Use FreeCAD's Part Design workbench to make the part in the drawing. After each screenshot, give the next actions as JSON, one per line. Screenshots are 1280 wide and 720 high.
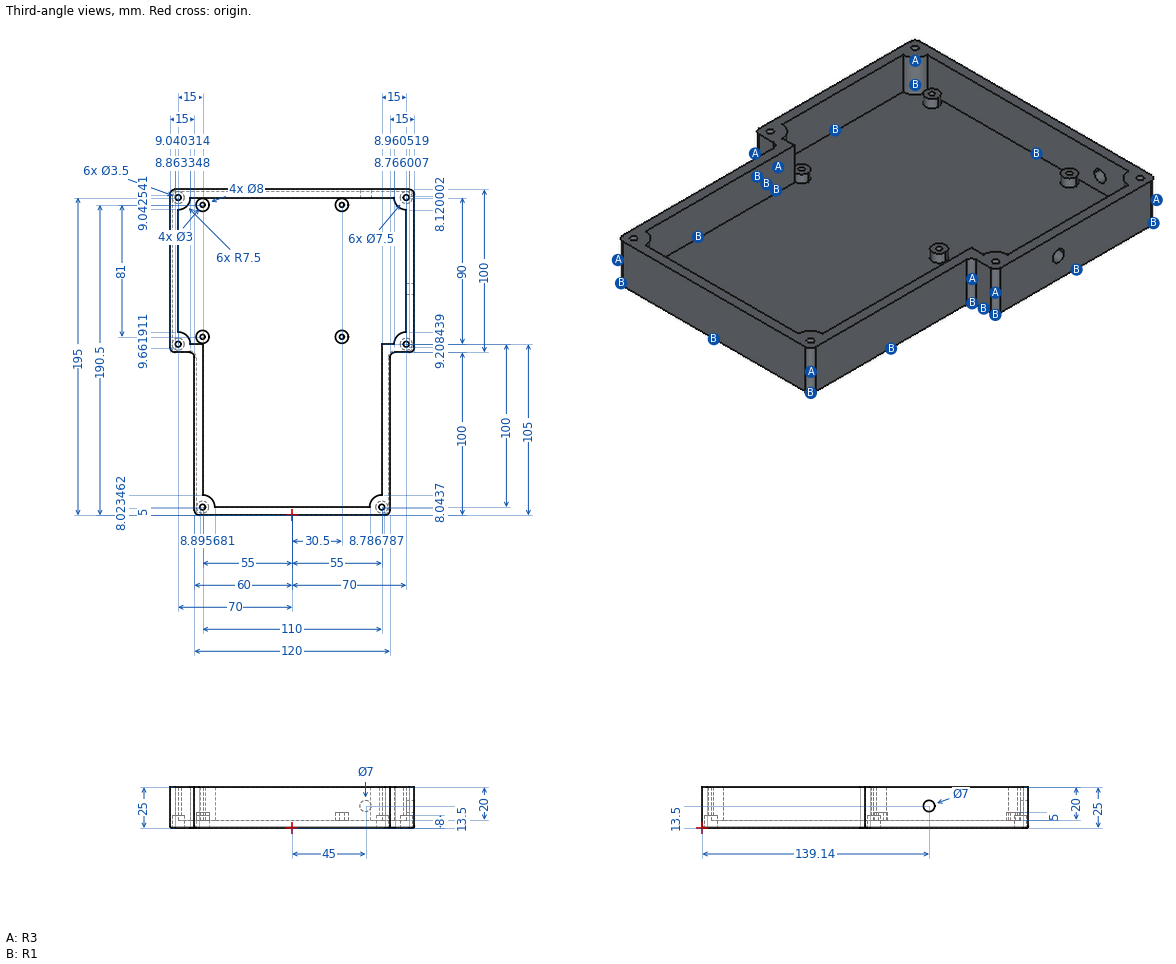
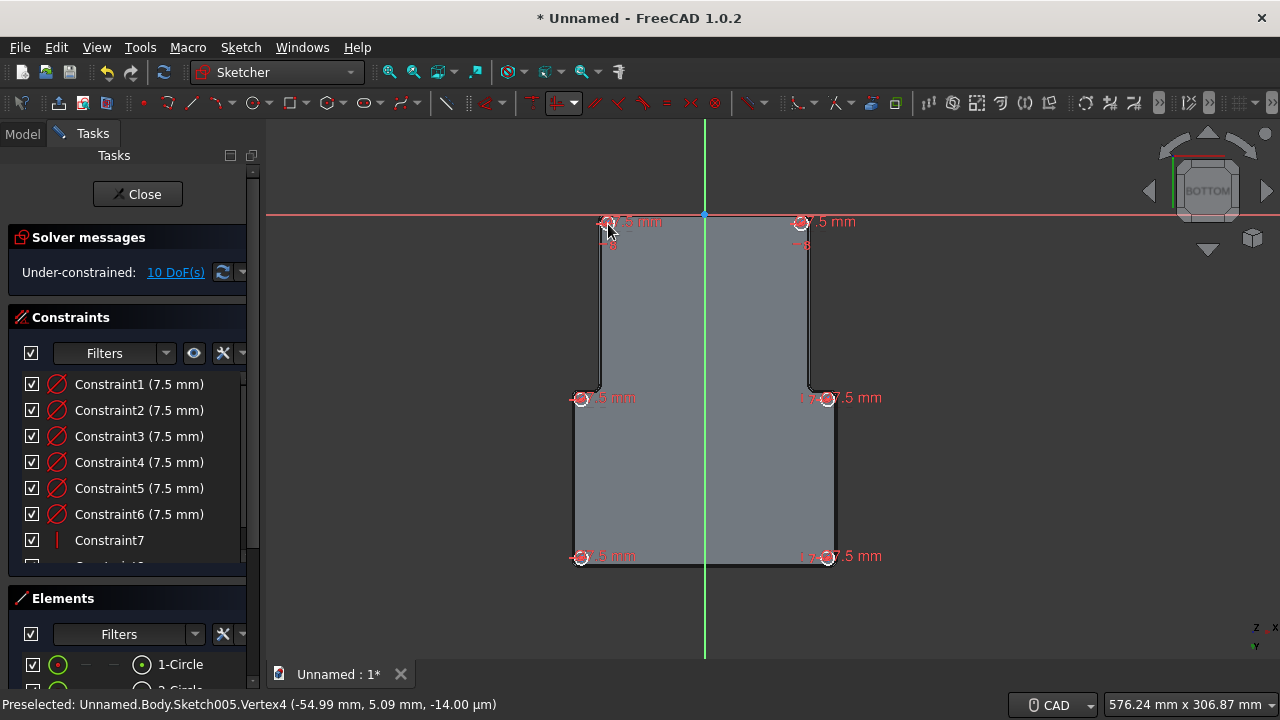
{"action": "left_click", "coordinate": [828, 400]}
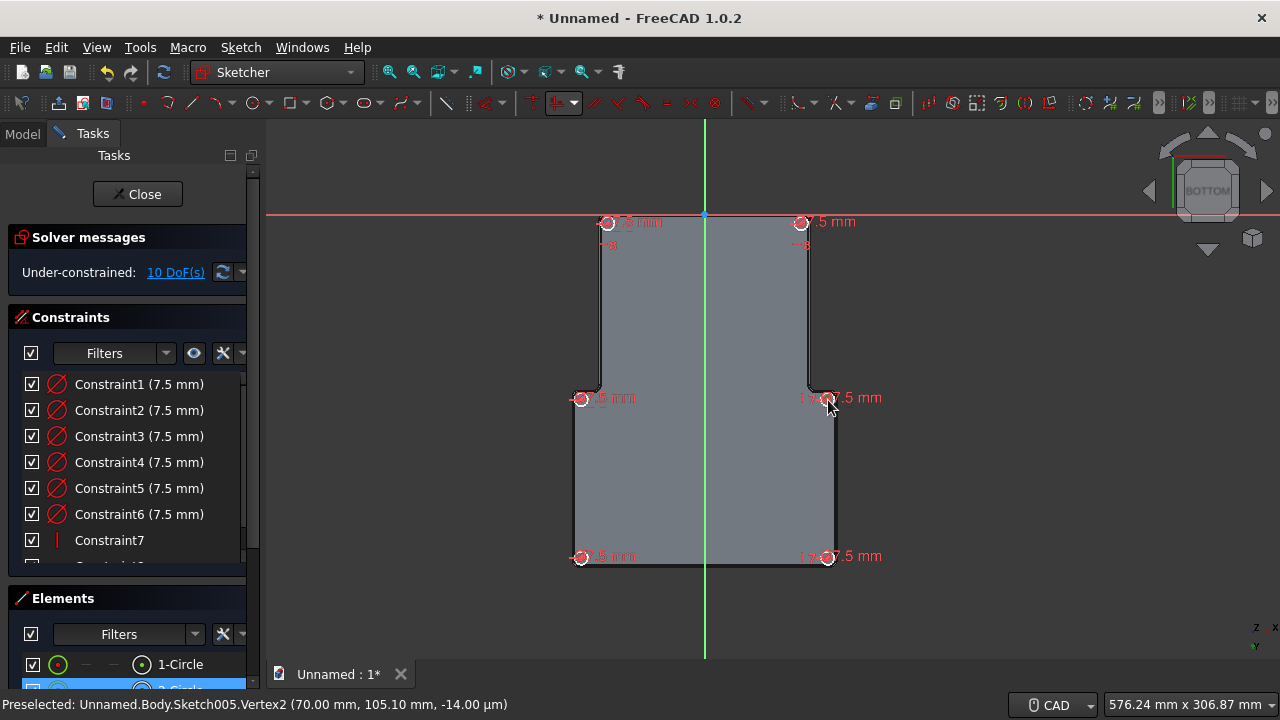
{"action": "left_click", "coordinate": [581, 400]}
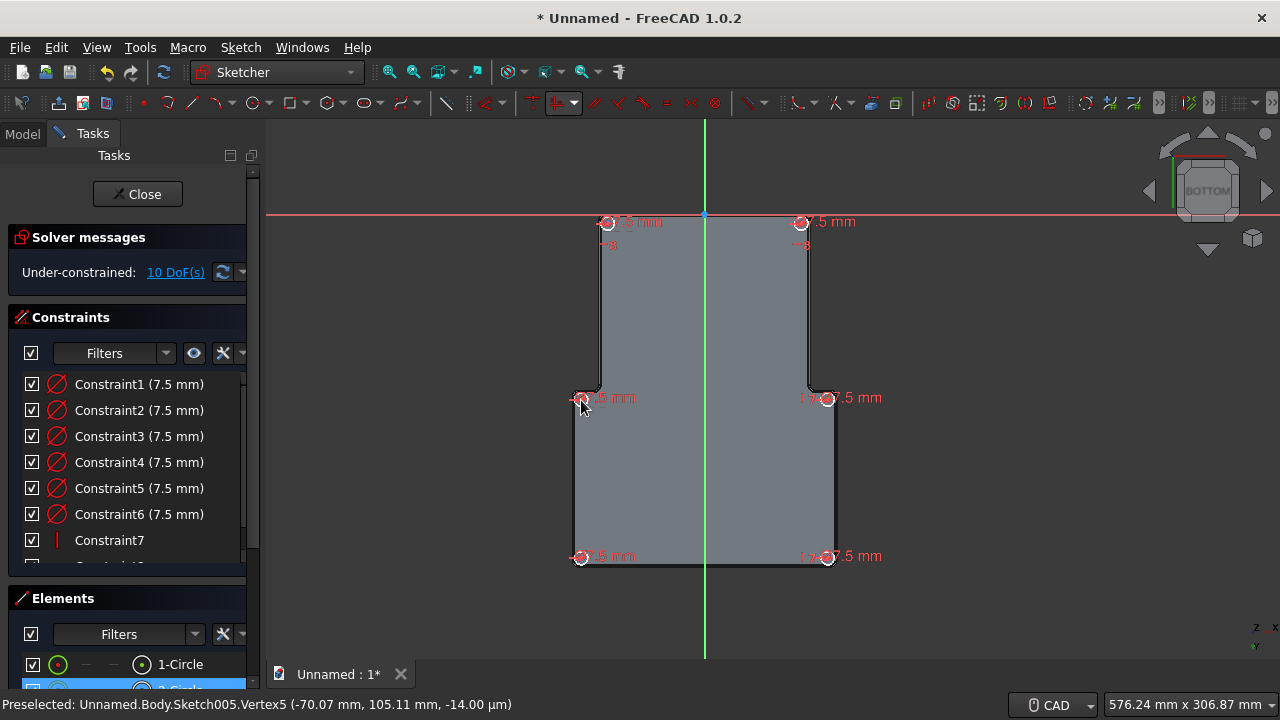
{"action": "key", "text": "h"}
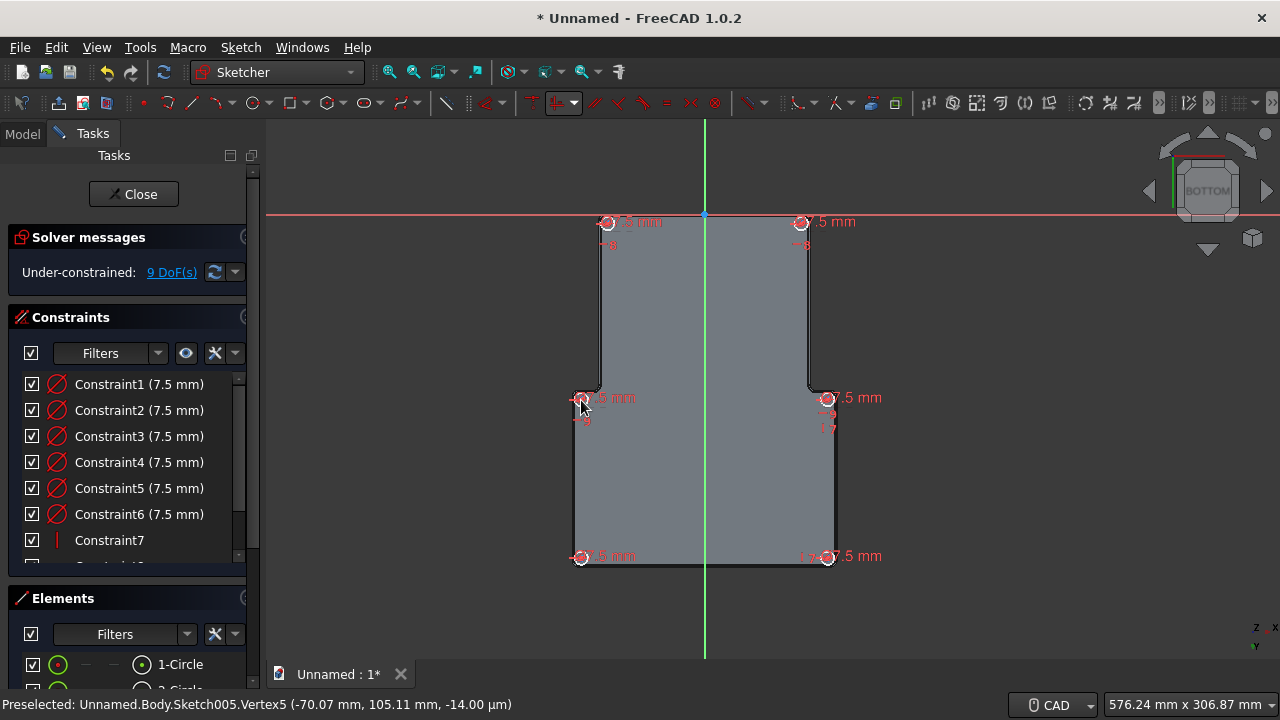
{"action": "left_click", "coordinate": [581, 400]}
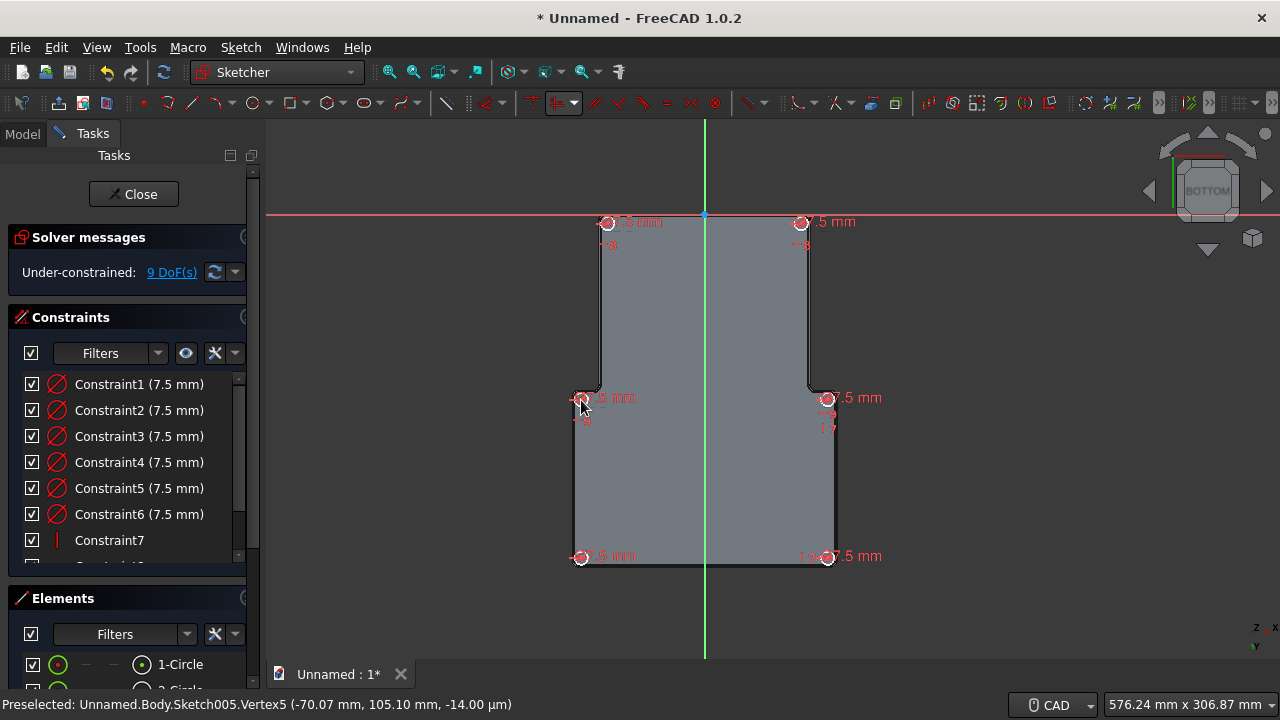
{"action": "left_click", "coordinate": [581, 558]}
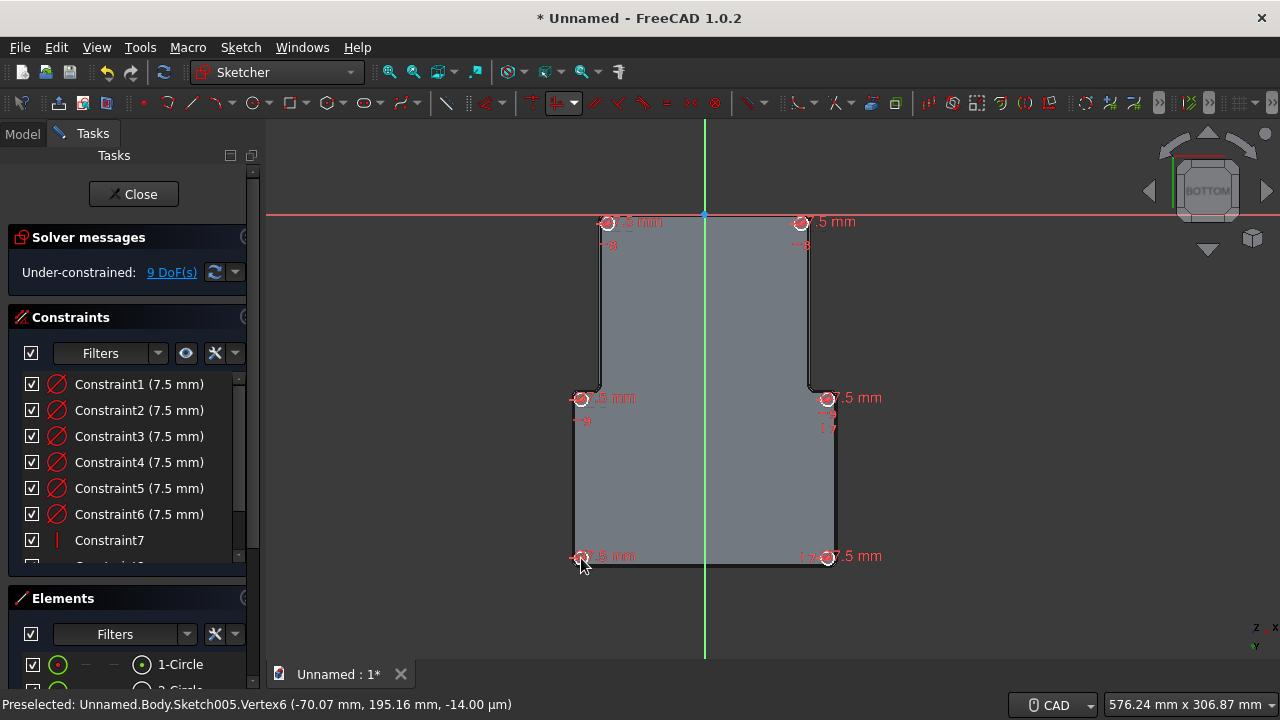
{"action": "key", "text": "v"}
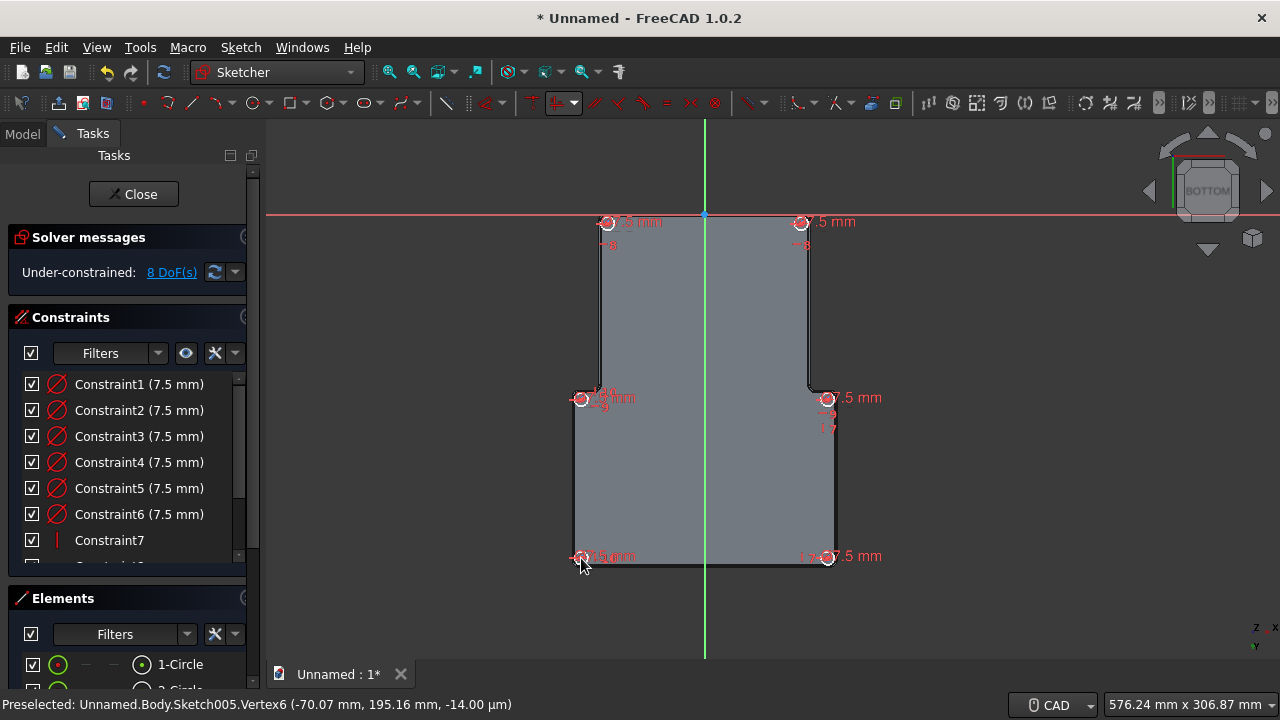
{"action": "left_click", "coordinate": [828, 558]}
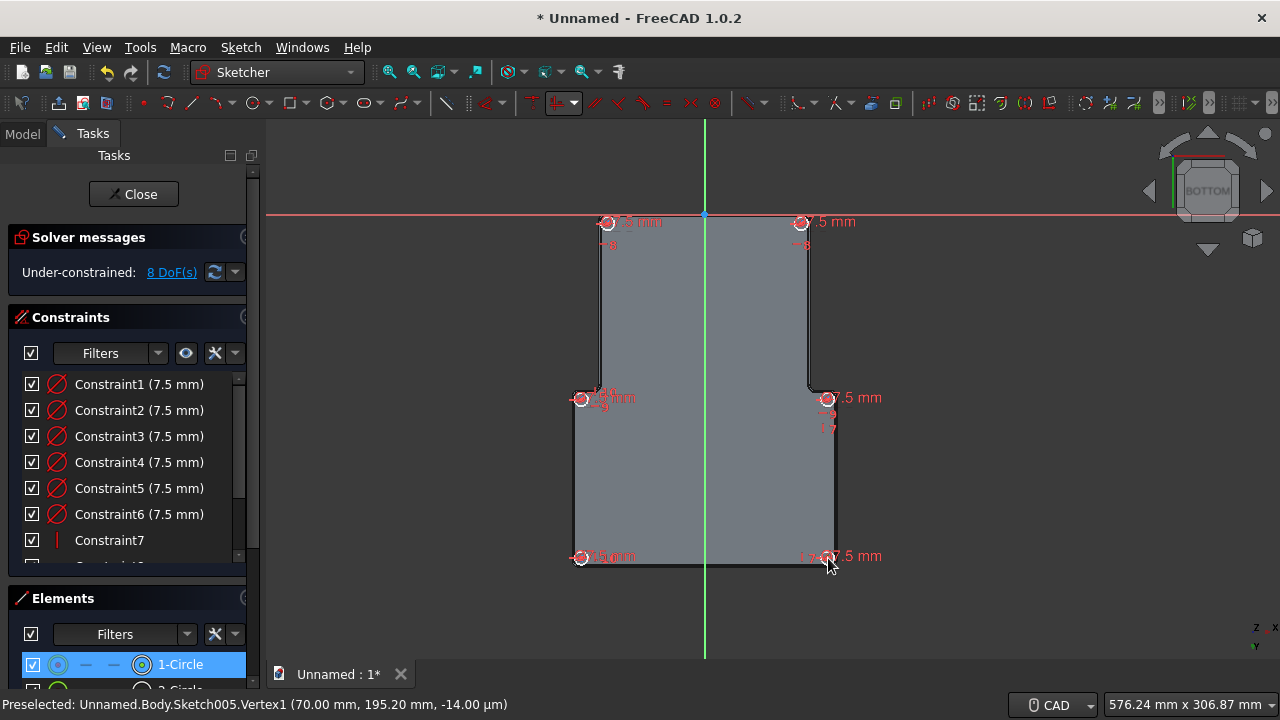
{"action": "left_click", "coordinate": [581, 558]}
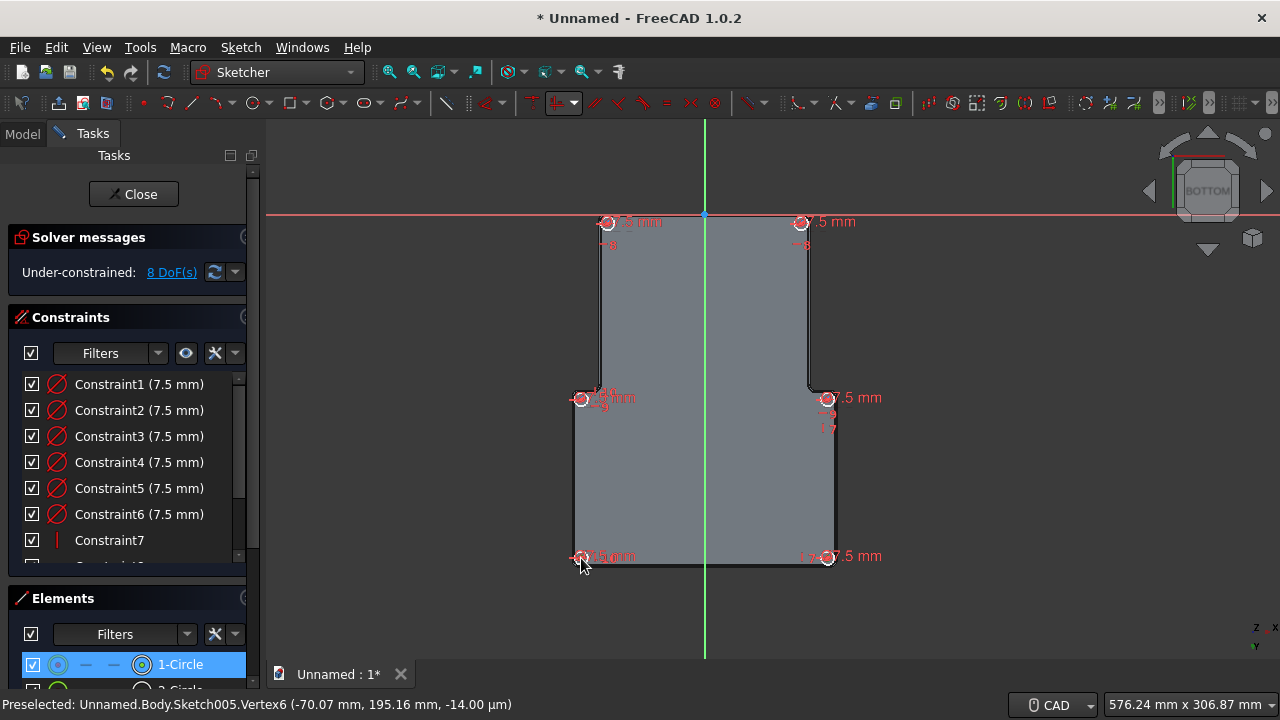
{"action": "key", "text": "h"}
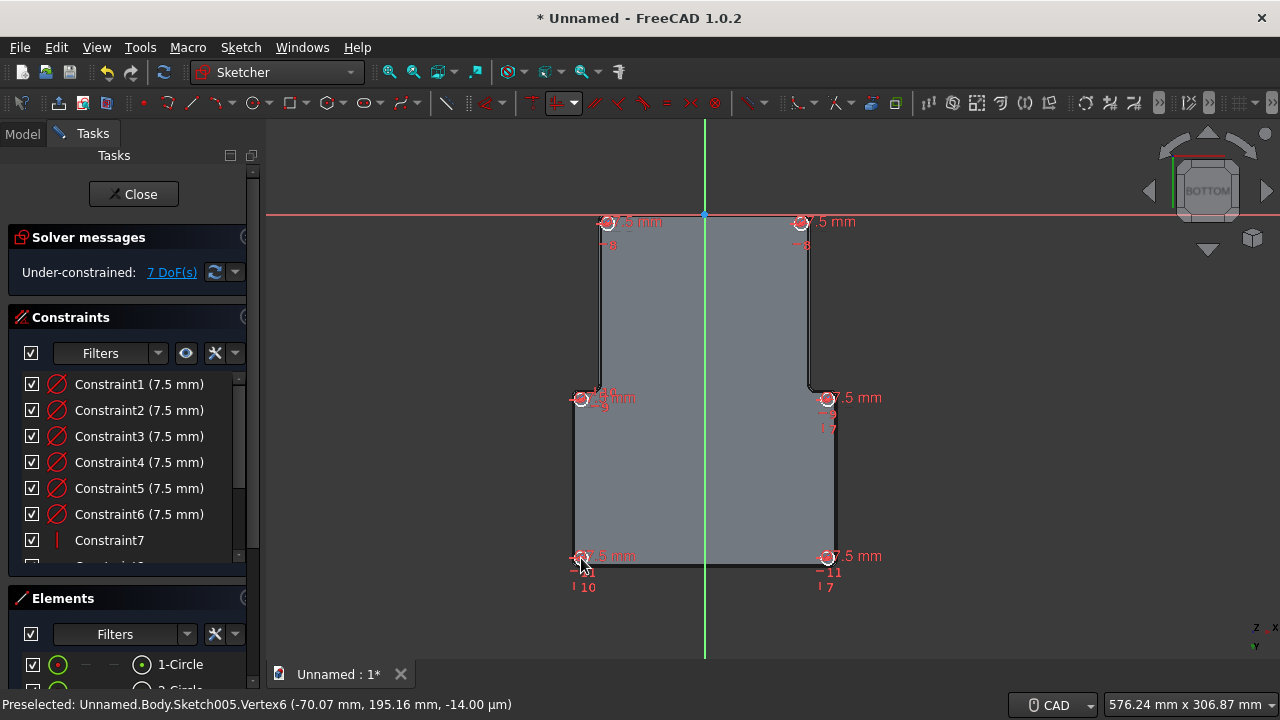
{"action": "left_click", "coordinate": [486, 104]}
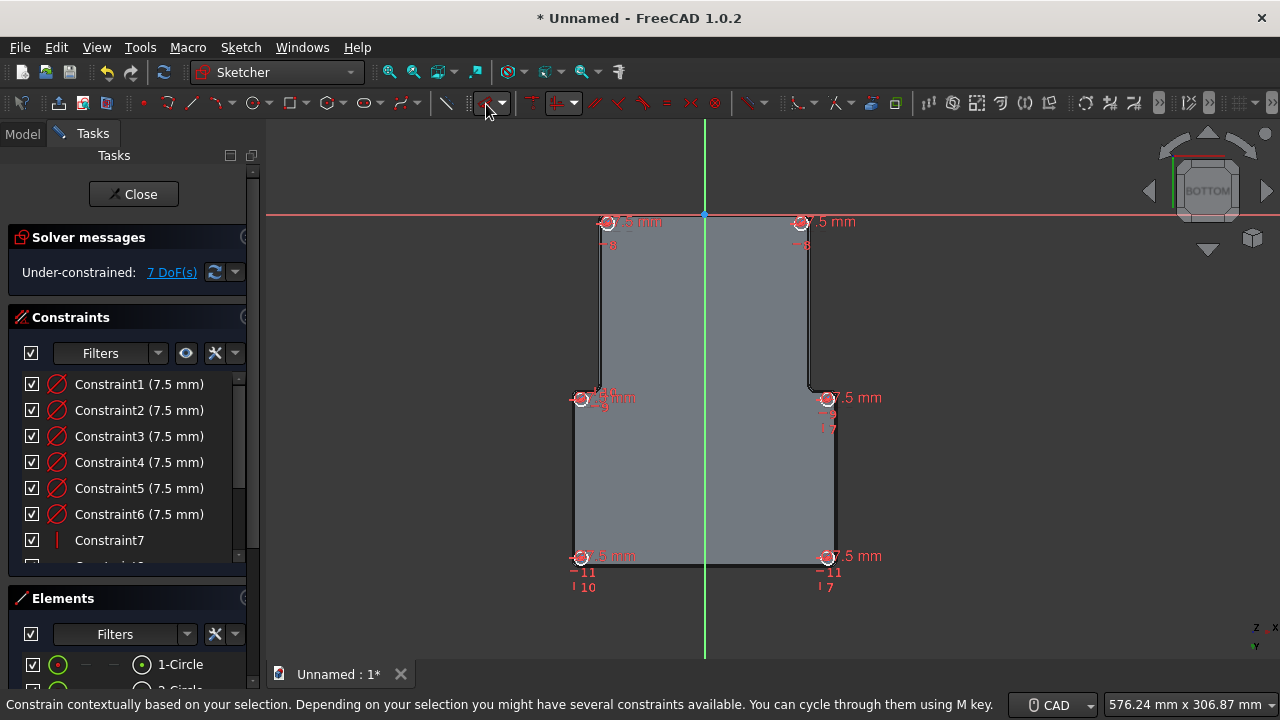
{"action": "scroll", "coordinate": [801, 224], "scroll_direction": "up", "scroll_amount": 8}